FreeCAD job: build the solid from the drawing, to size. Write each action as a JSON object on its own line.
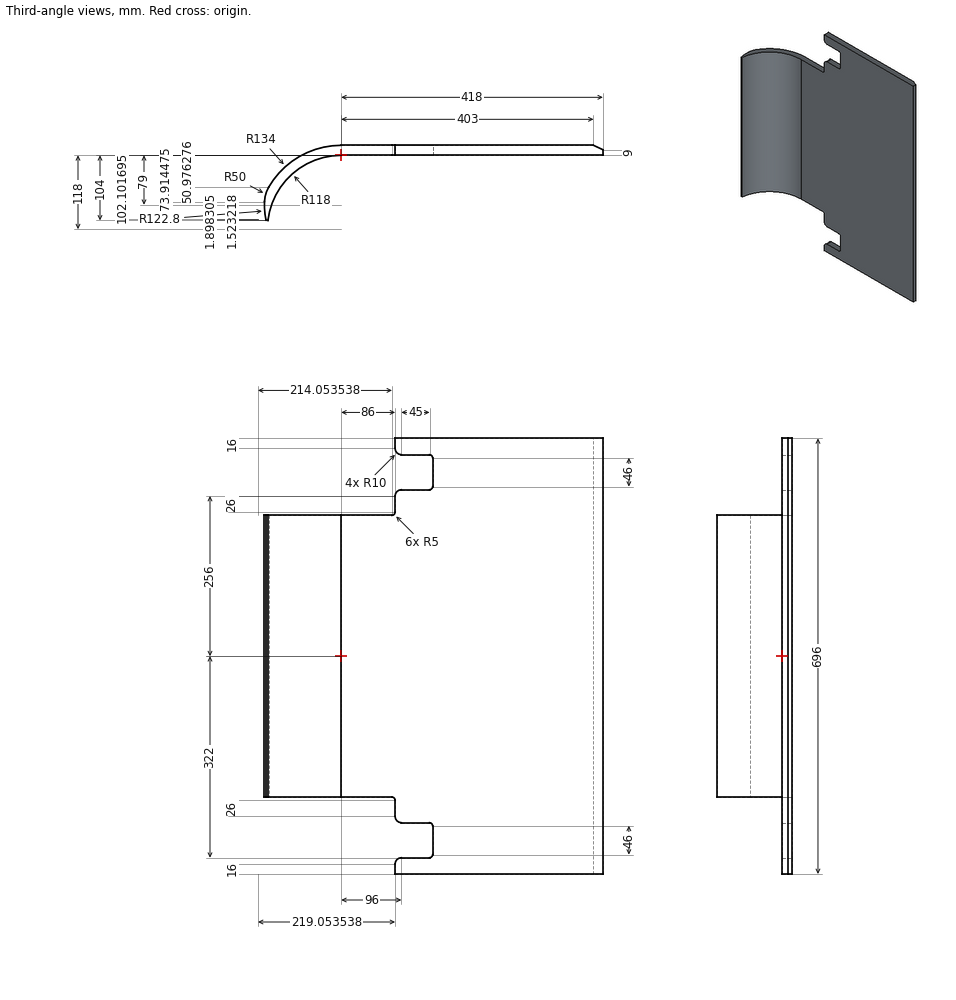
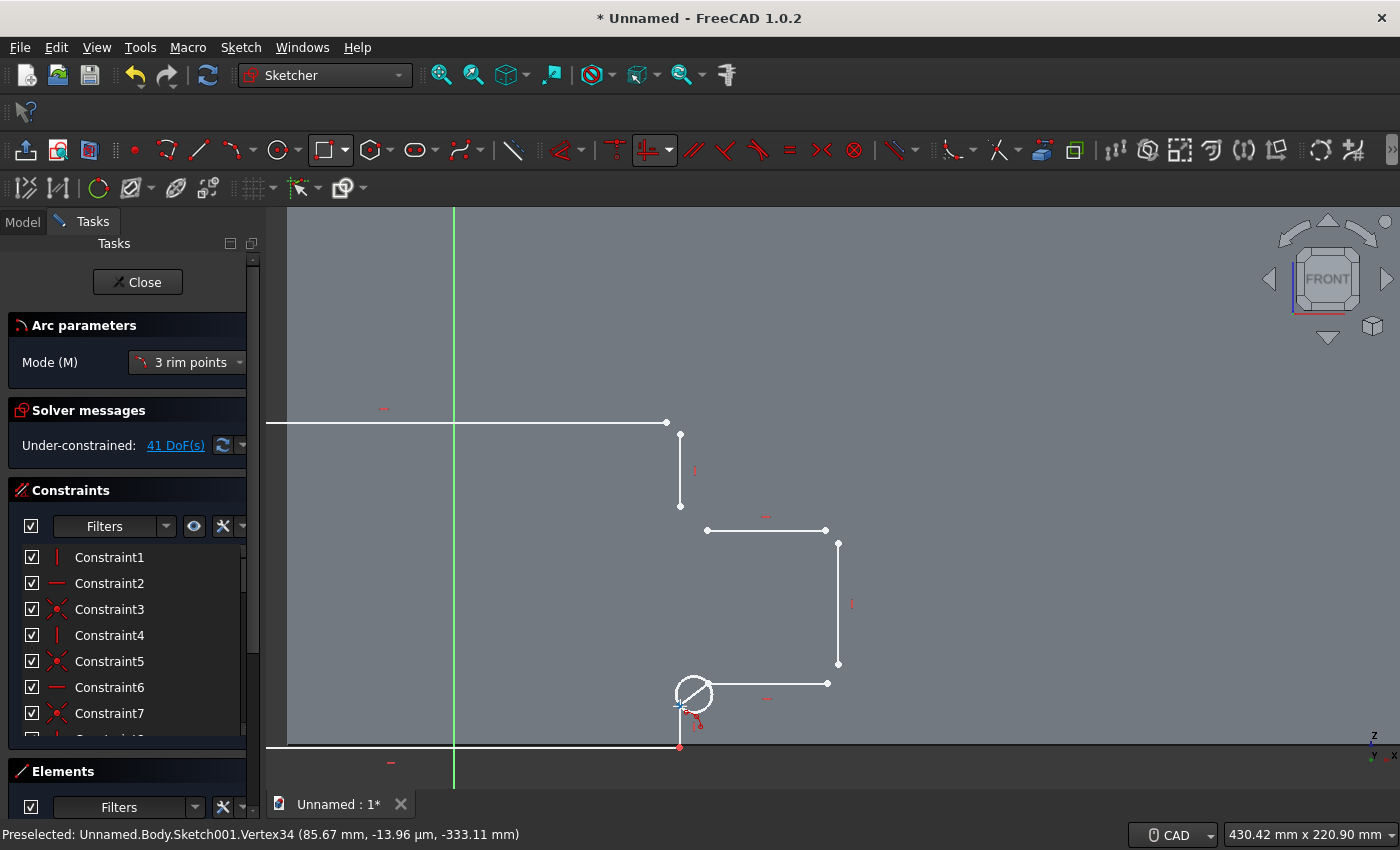
{"action": "scroll", "coordinate": [688, 684], "scroll_direction": "up", "scroll_amount": 4}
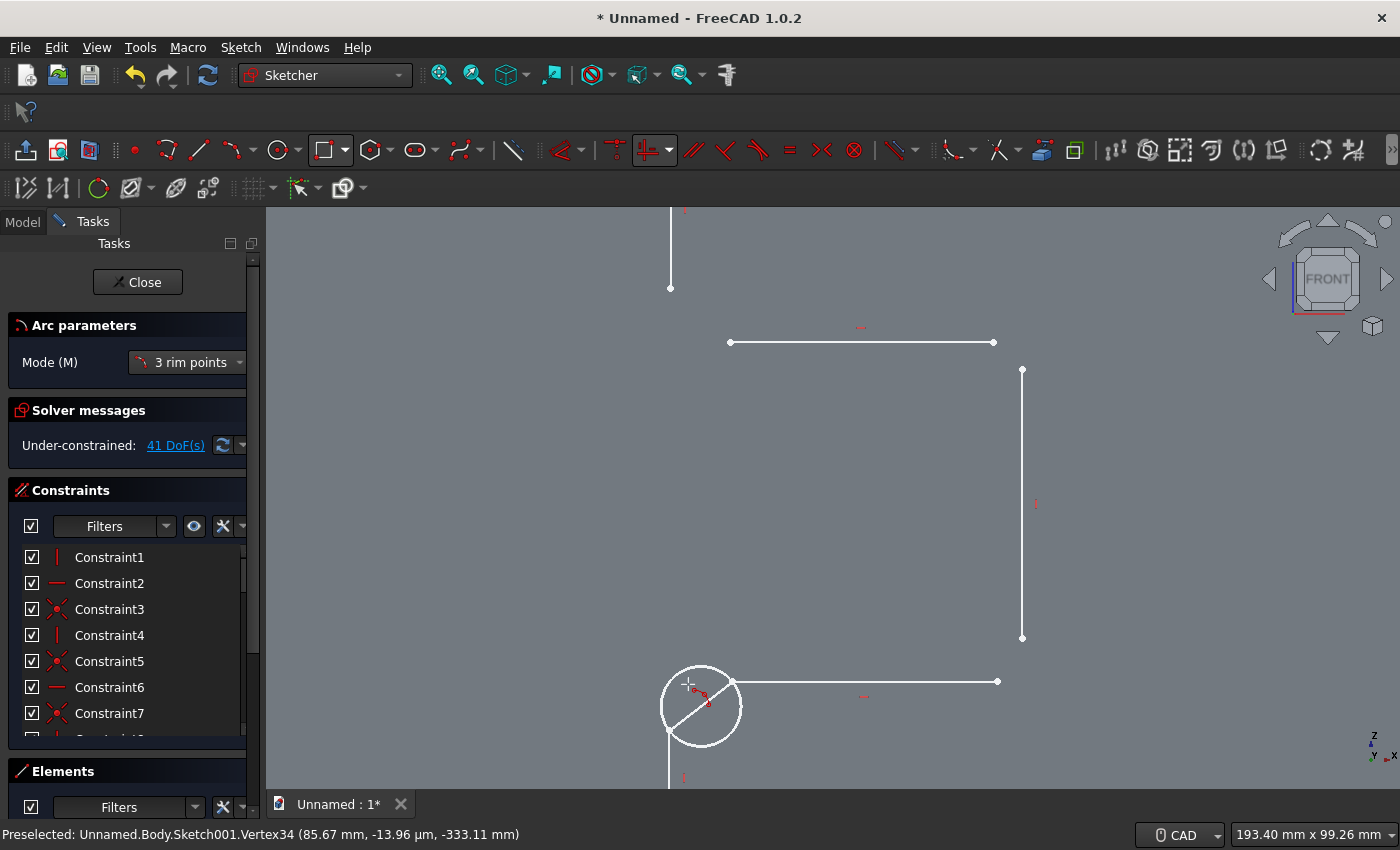
{"action": "left_click", "coordinate": [689, 683]}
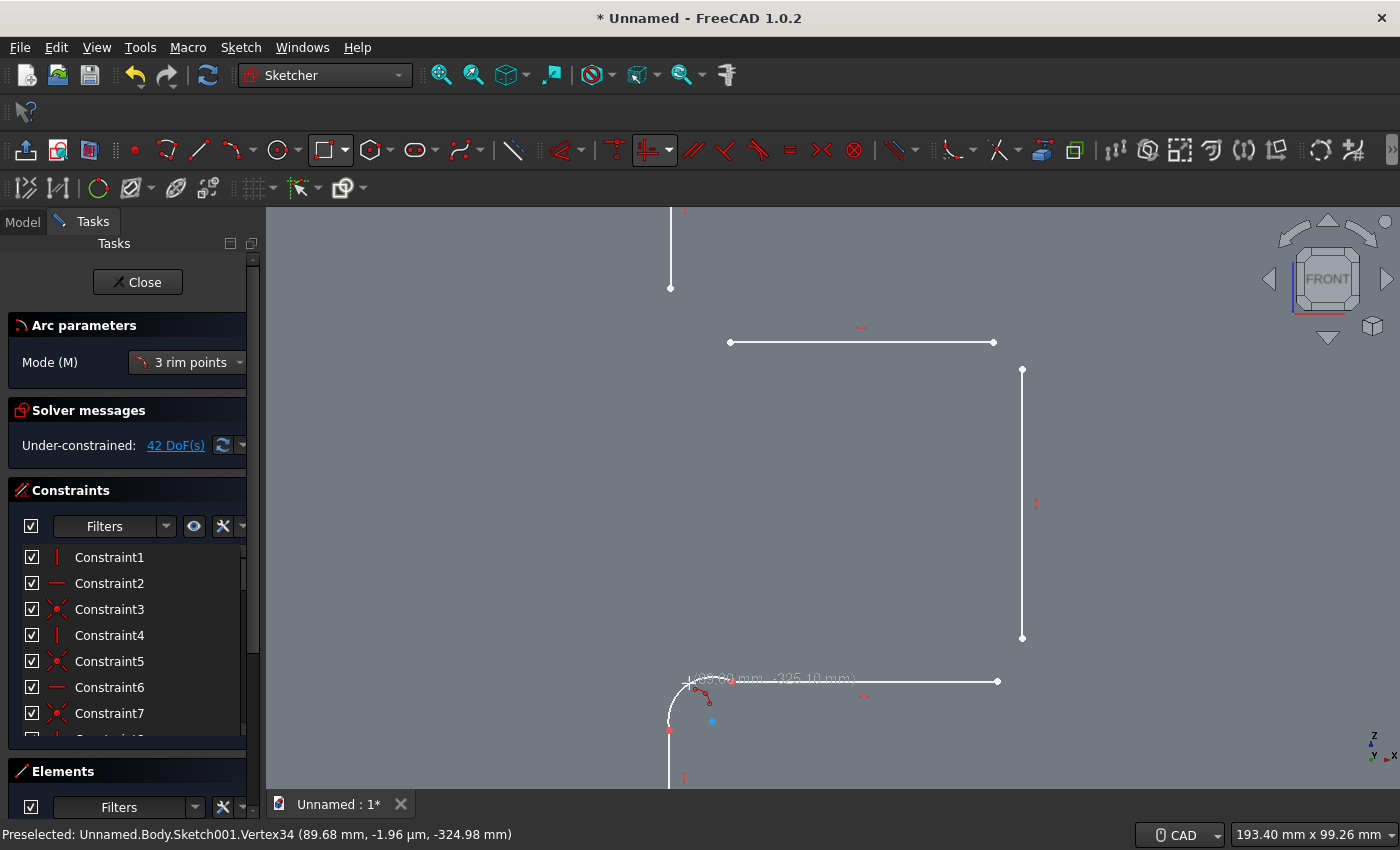
{"action": "scroll", "coordinate": [820, 670], "scroll_direction": "down", "scroll_amount": 12}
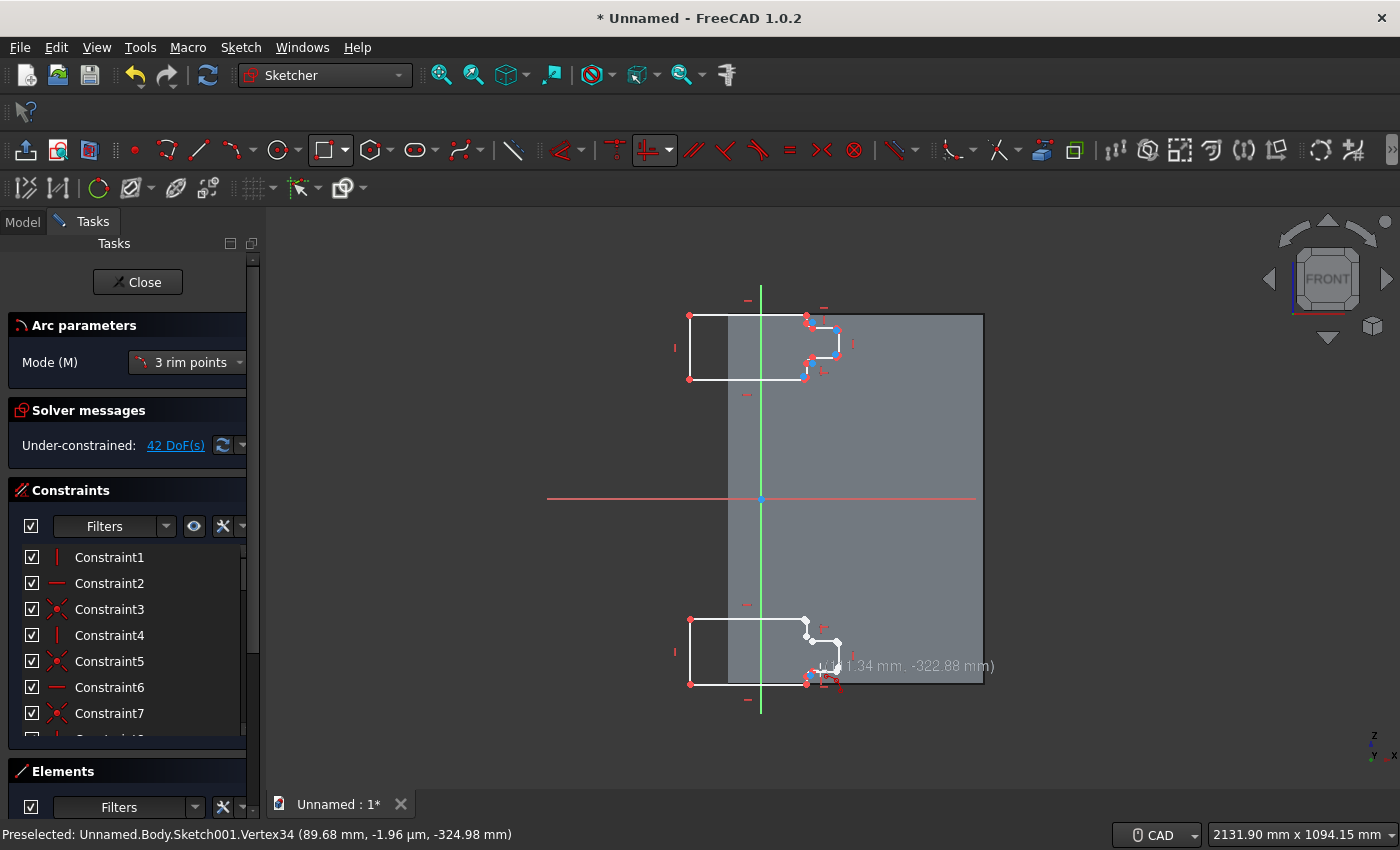
{"action": "scroll", "coordinate": [804, 619], "scroll_direction": "up", "scroll_amount": 8}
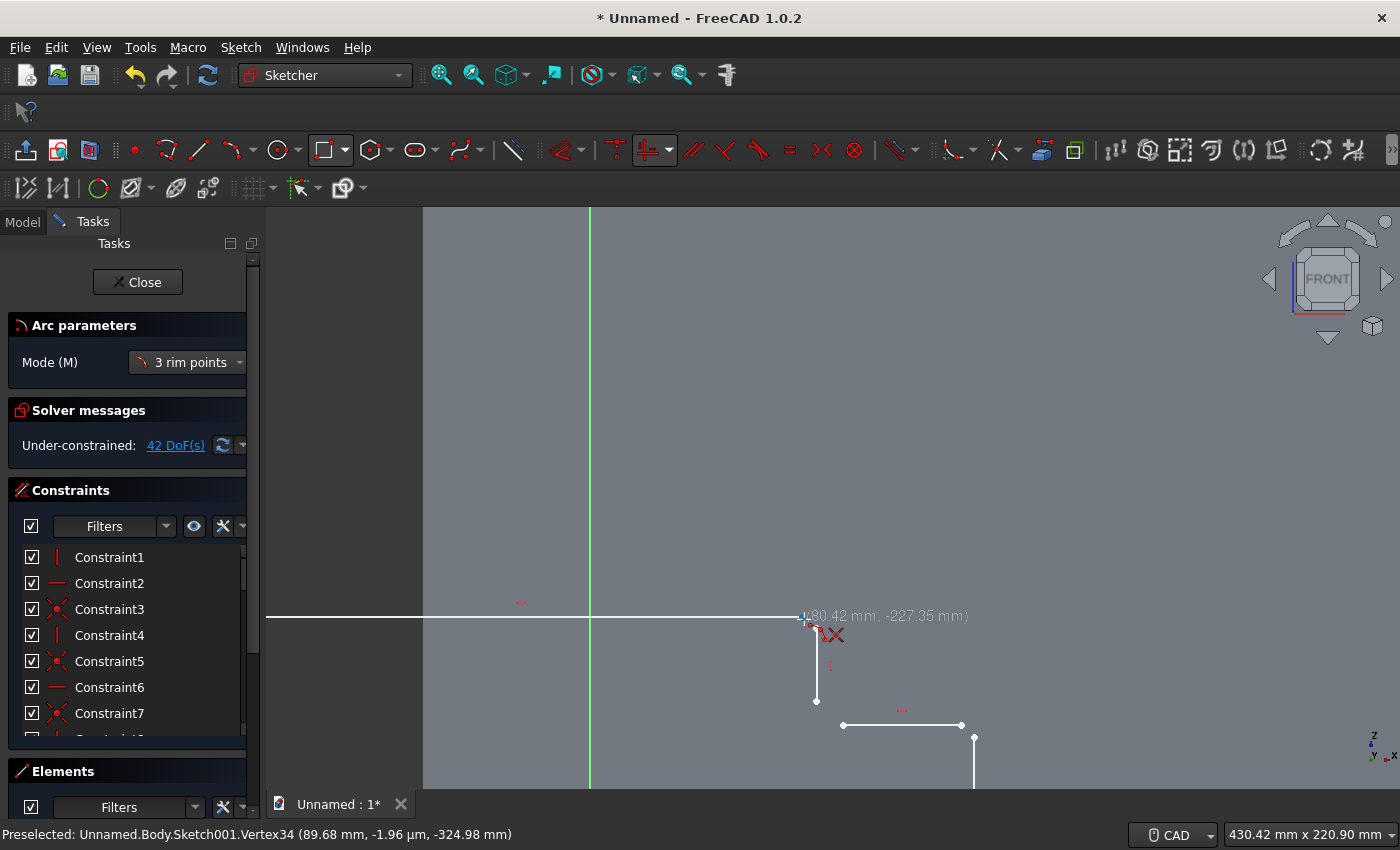
{"action": "left_click", "coordinate": [803, 617]}
{"action": "left_click", "coordinate": [817, 629]}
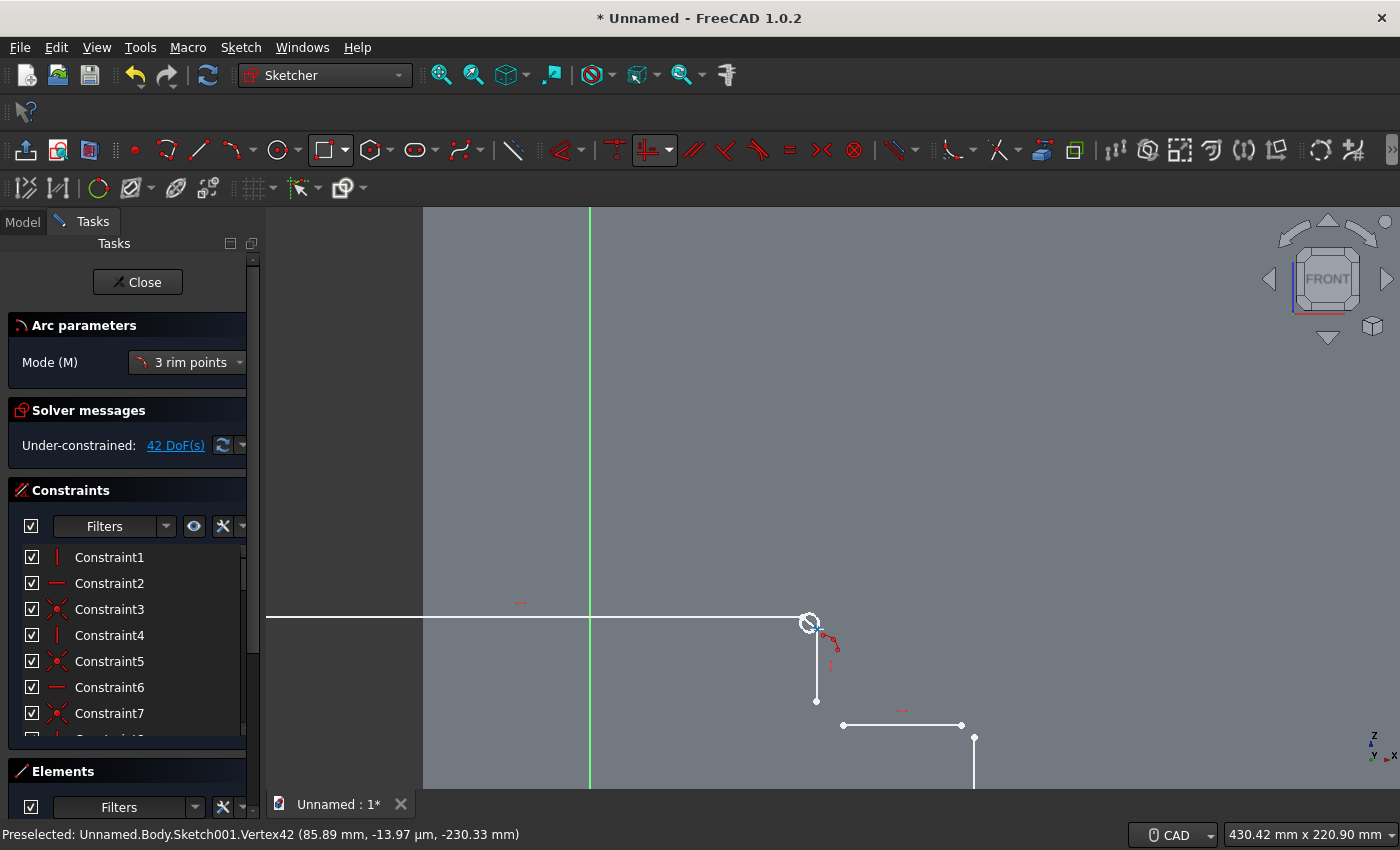
{"action": "scroll", "coordinate": [813, 619], "scroll_direction": "up", "scroll_amount": 8}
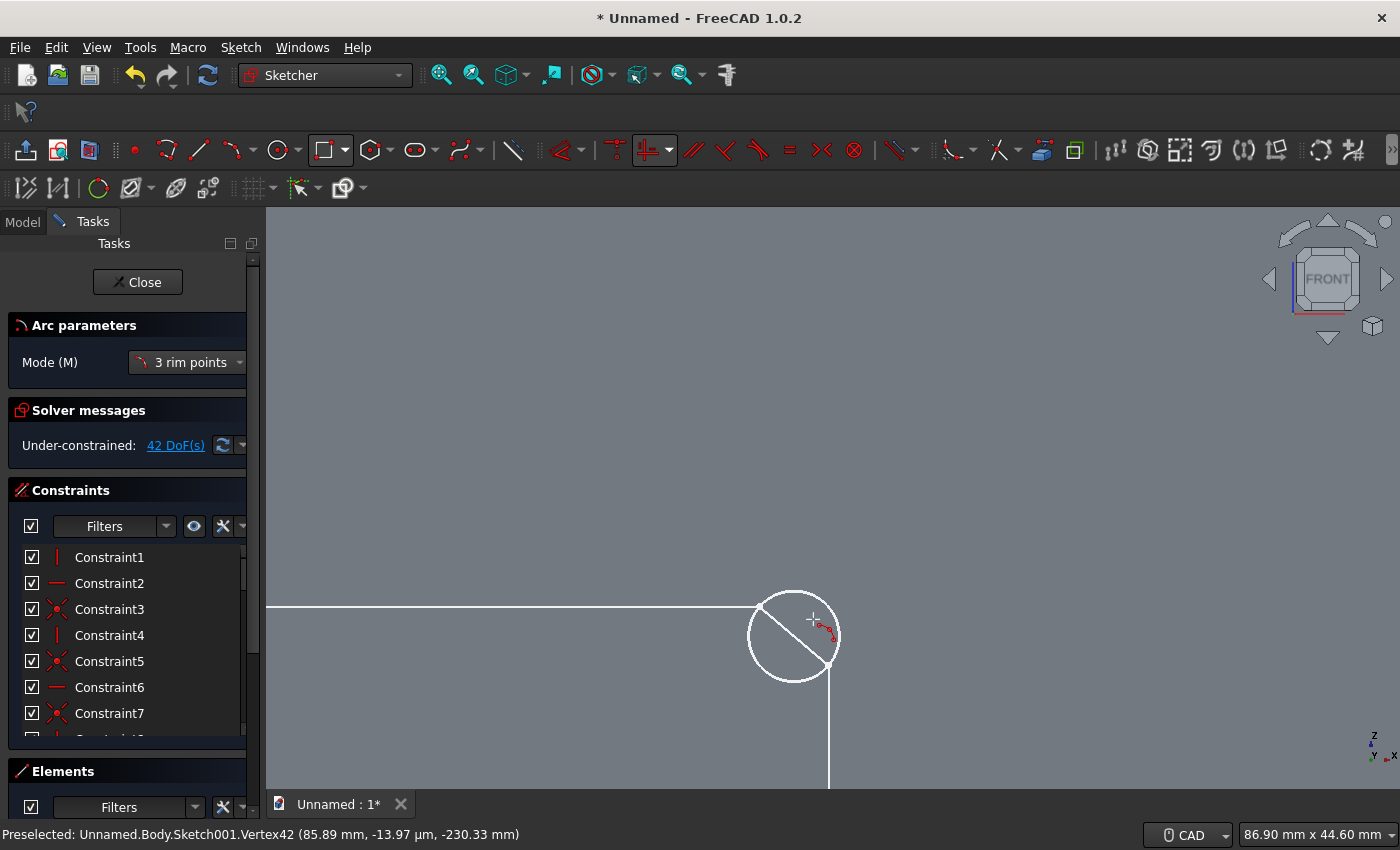
{"action": "left_click", "coordinate": [811, 615]}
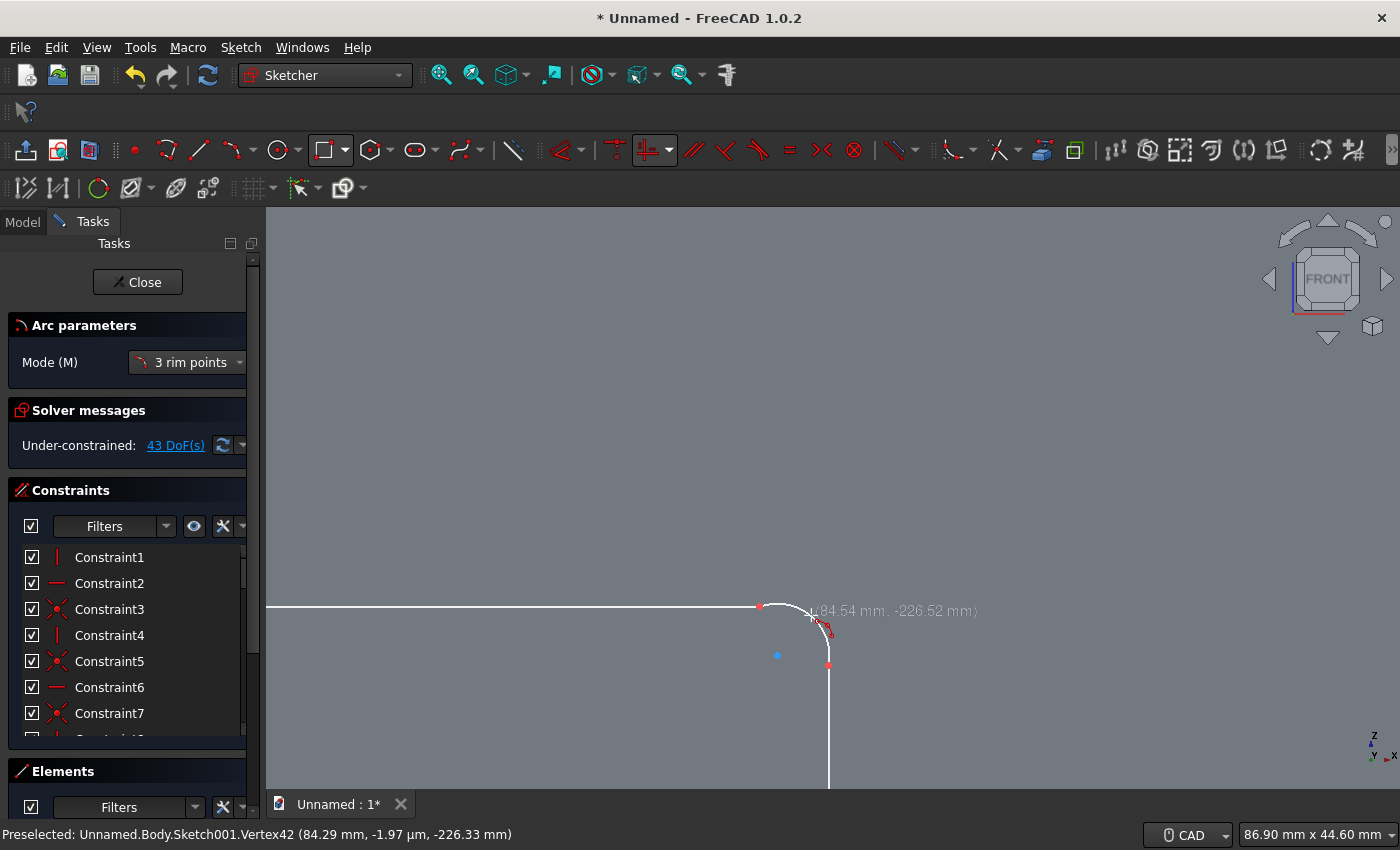
{"action": "scroll", "coordinate": [815, 647], "scroll_direction": "down", "scroll_amount": 15}